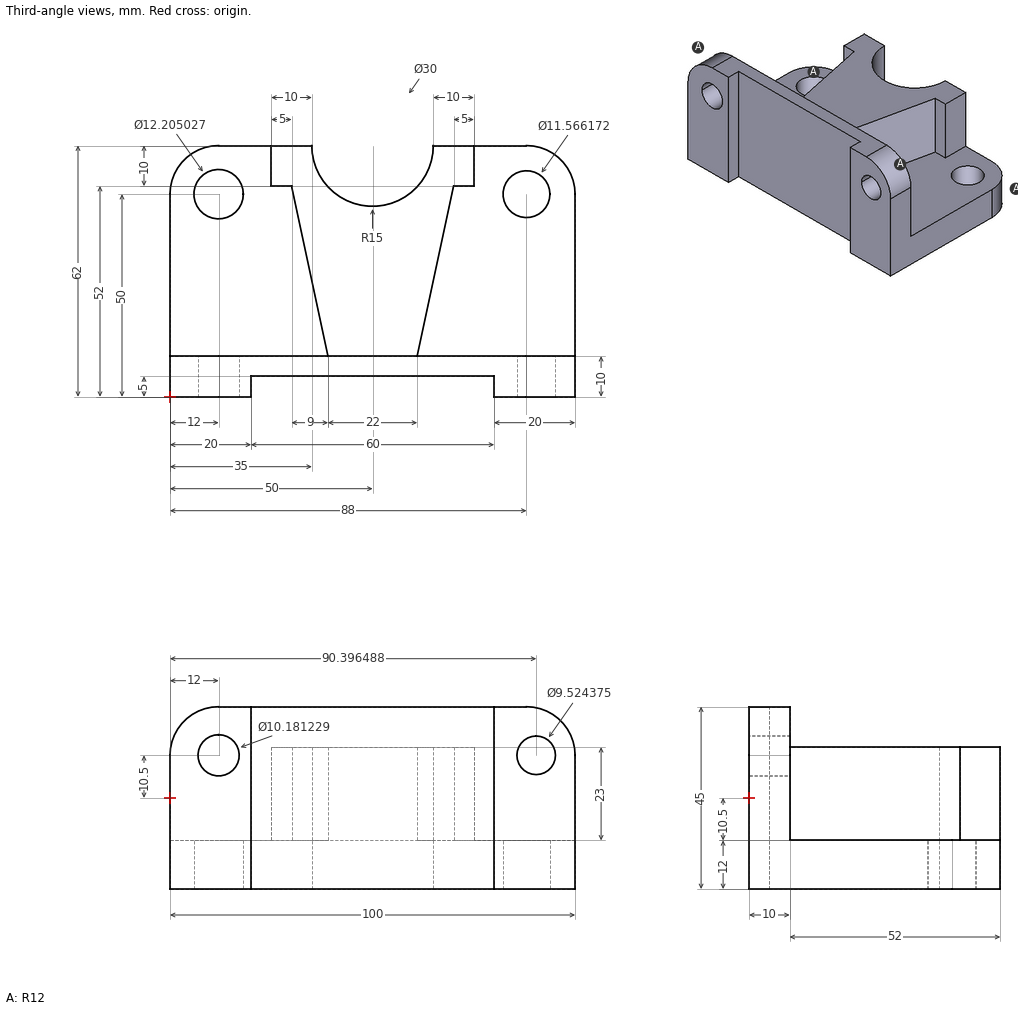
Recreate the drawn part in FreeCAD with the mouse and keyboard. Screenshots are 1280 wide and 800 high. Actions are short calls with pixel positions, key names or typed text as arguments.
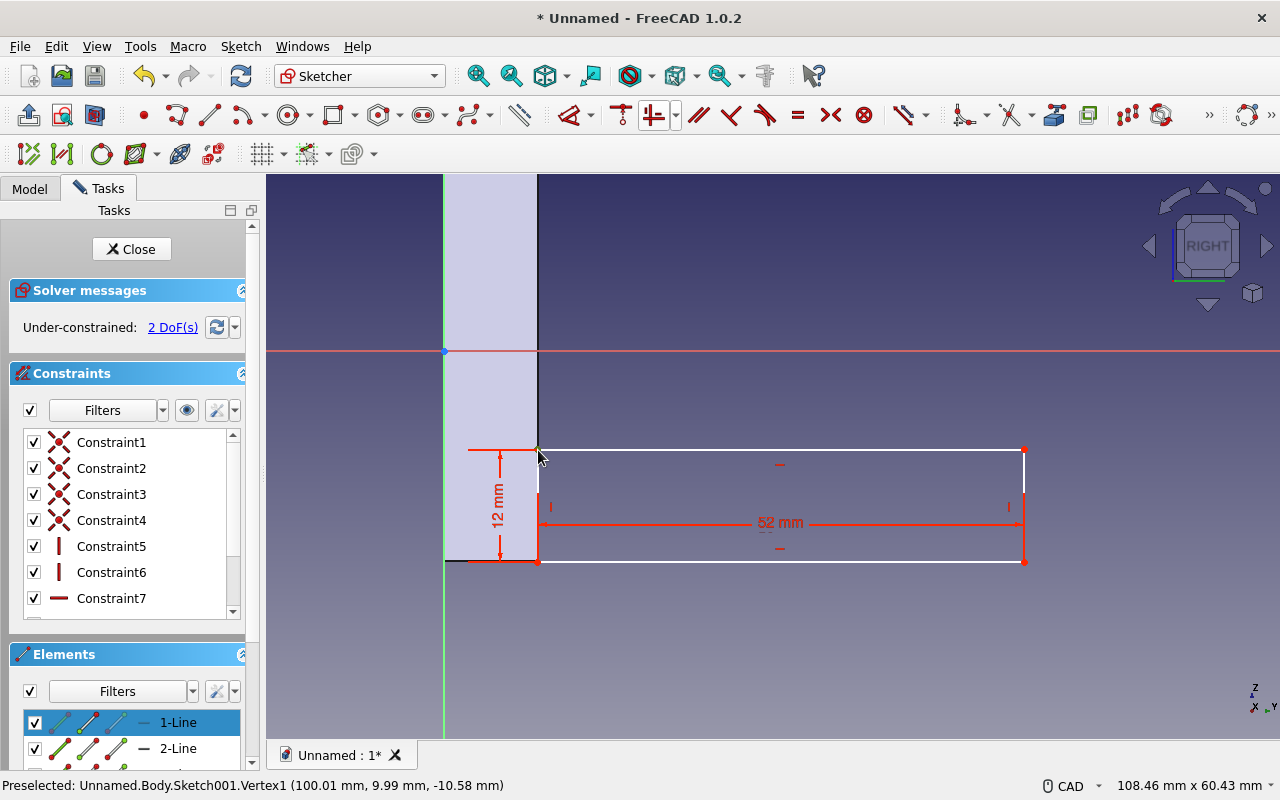
key(l)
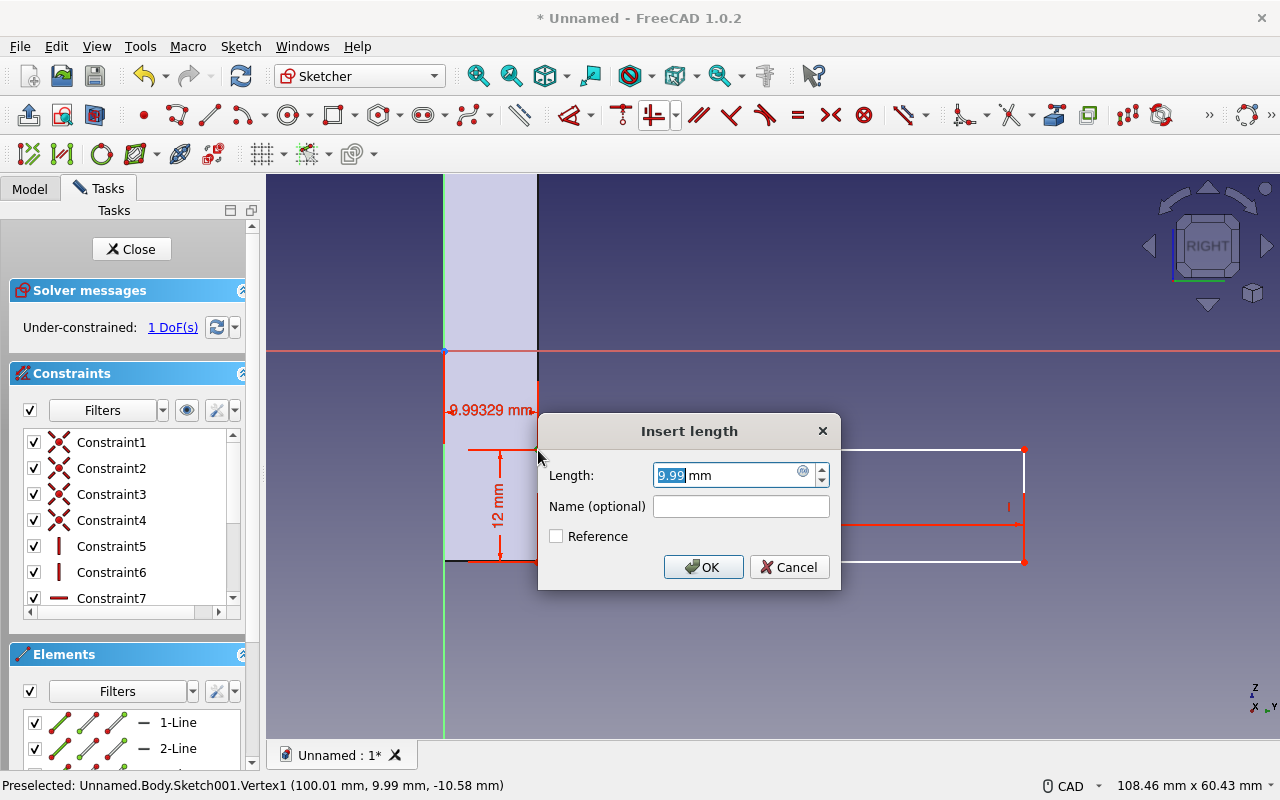
text(10)
key(Return)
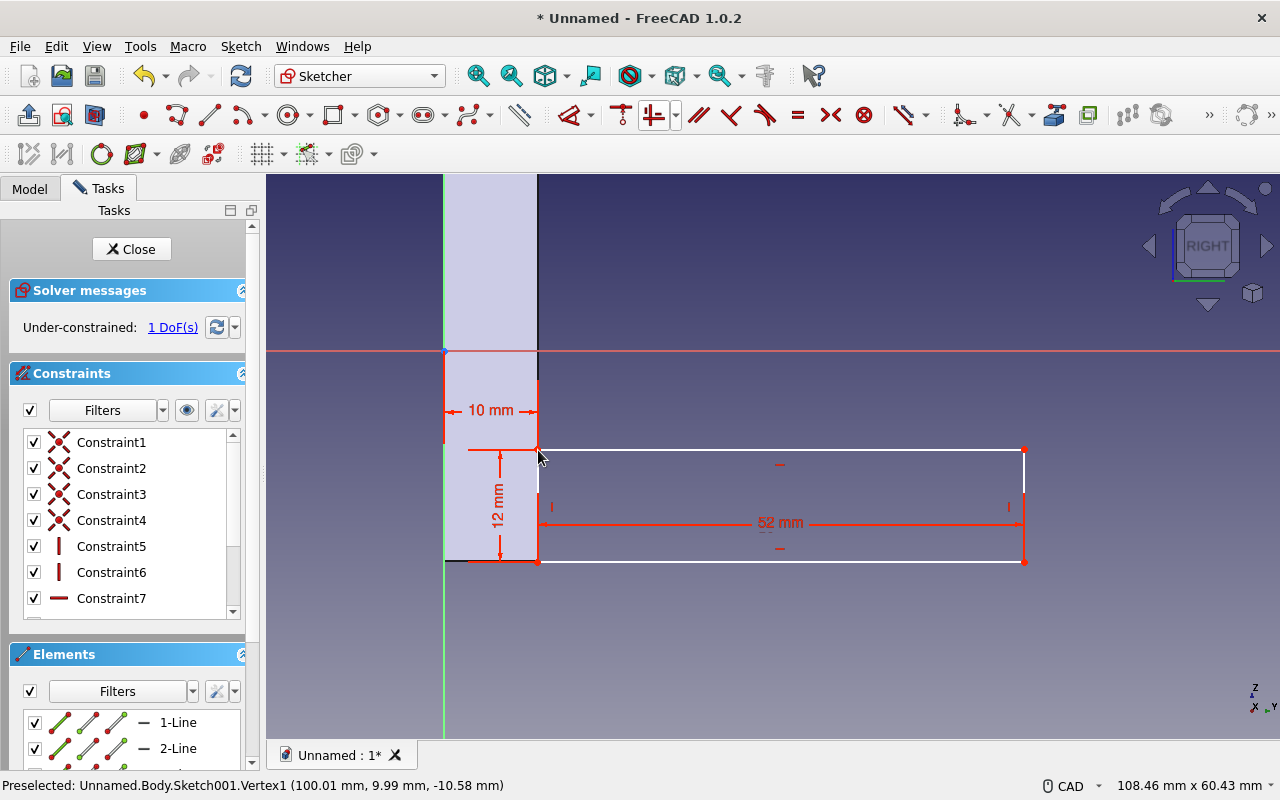
click(538, 450)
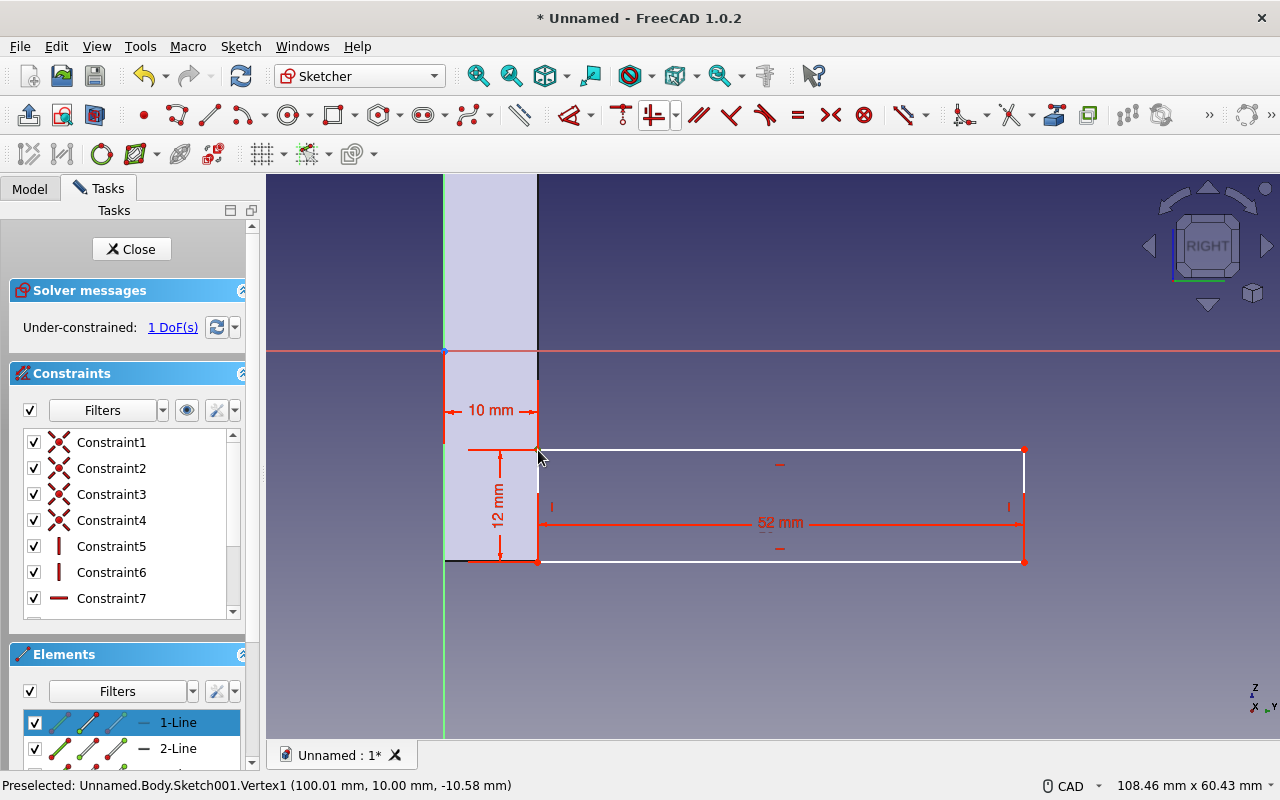
key(i)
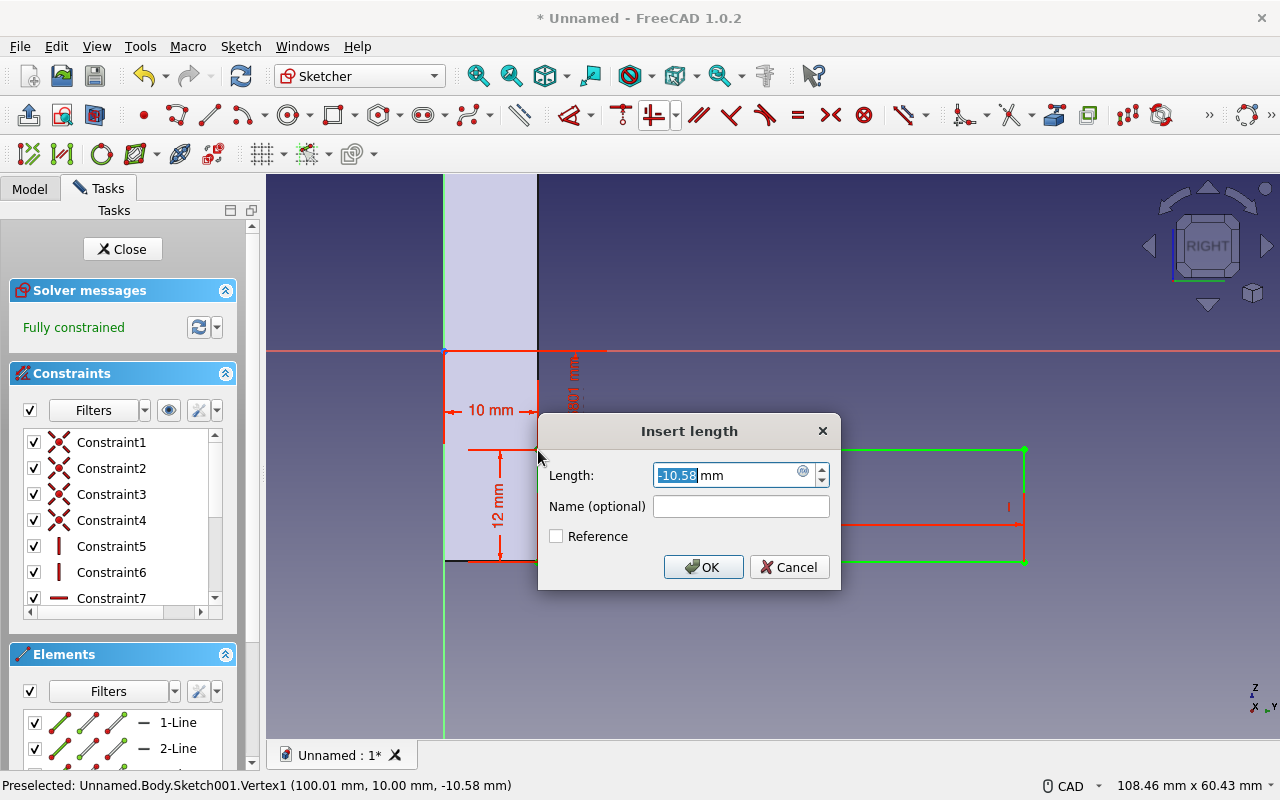
text(-10.5)
key(Return)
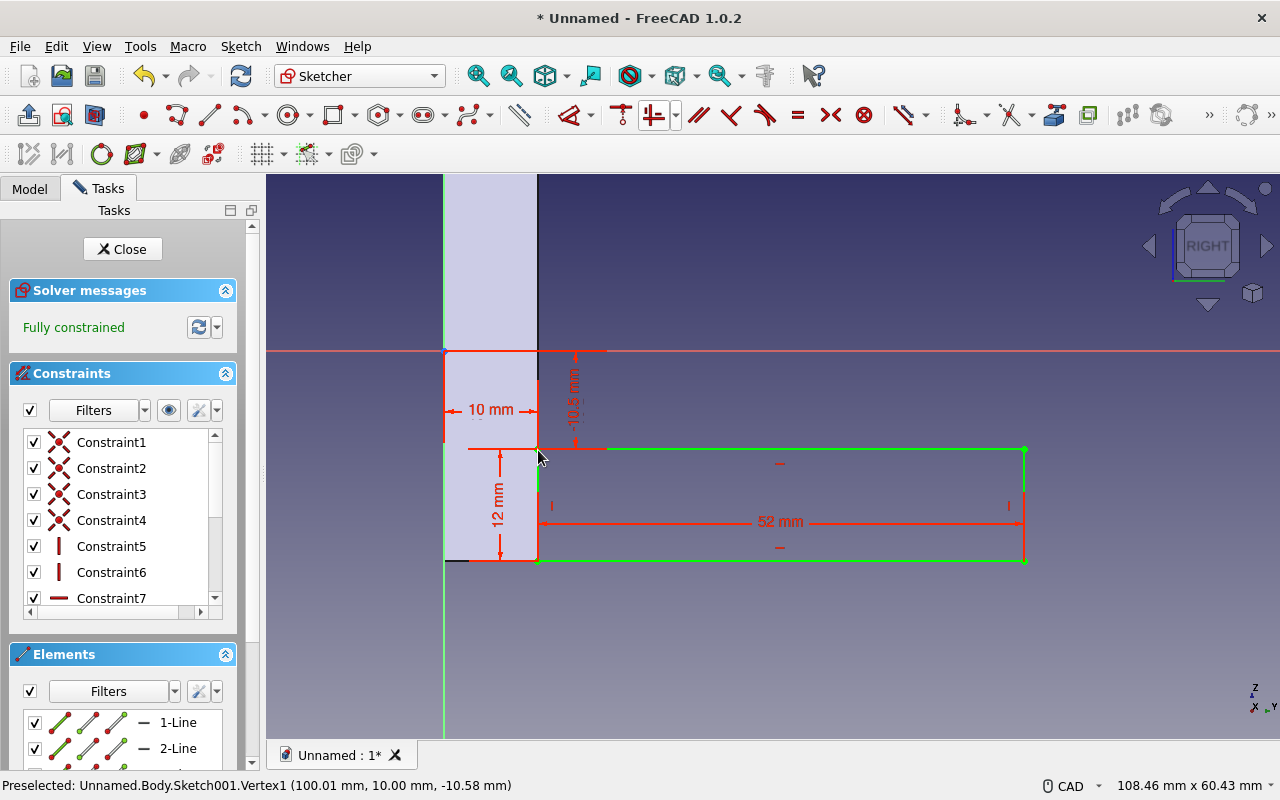
click(123, 249)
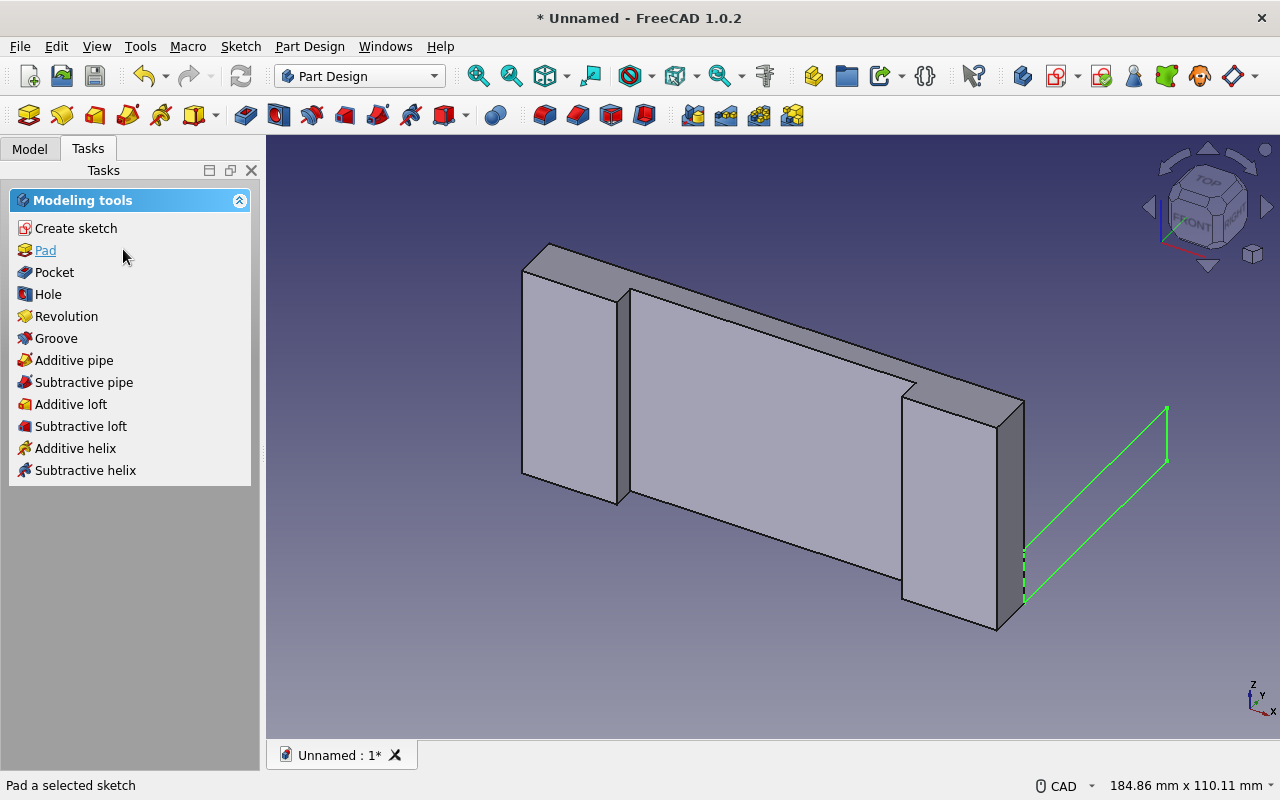
click(29, 116)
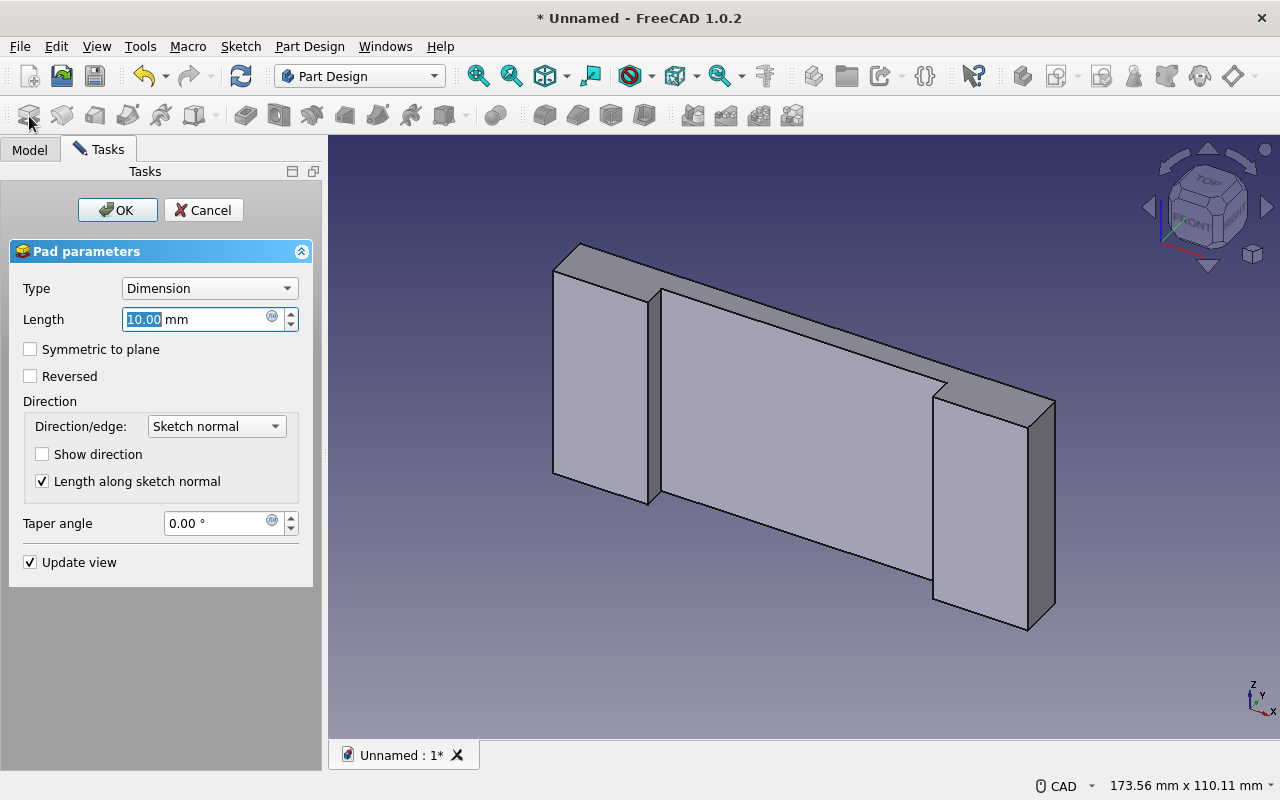
text(100)
key(Tab)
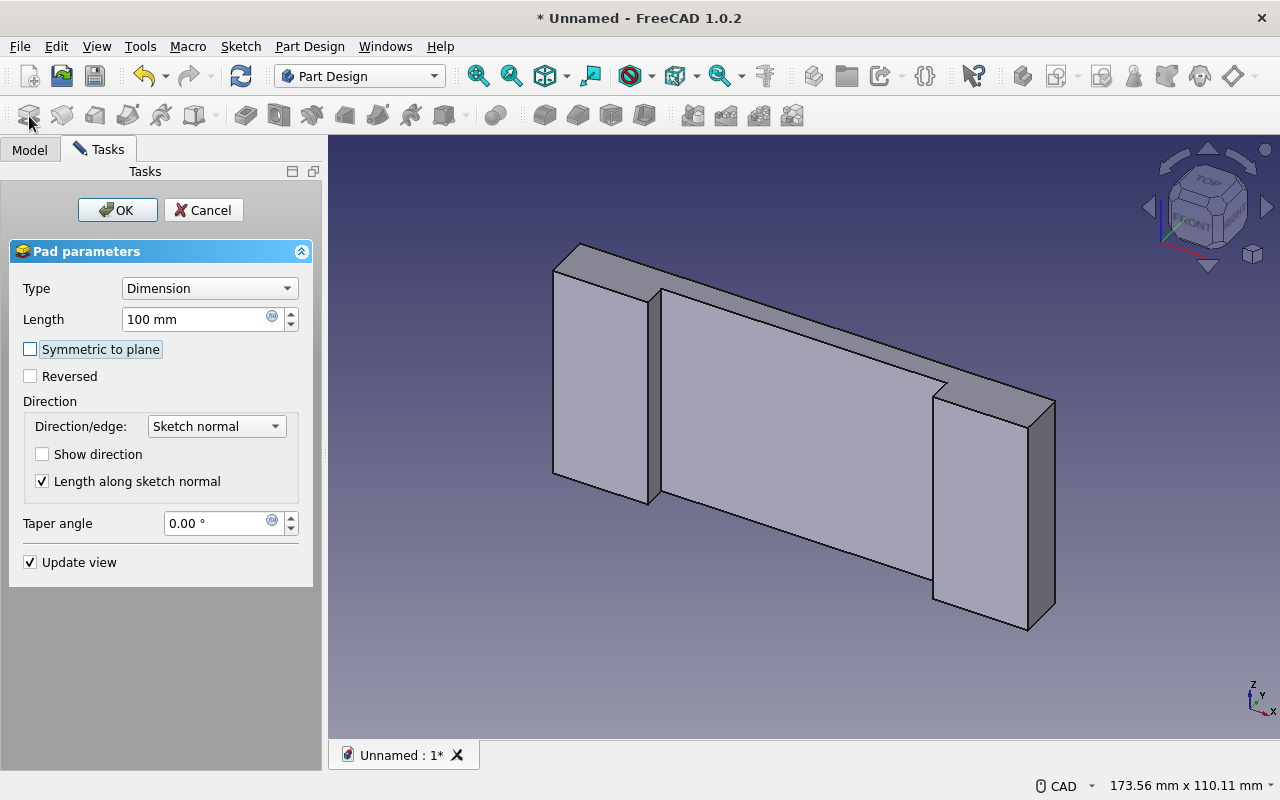
click(31, 376)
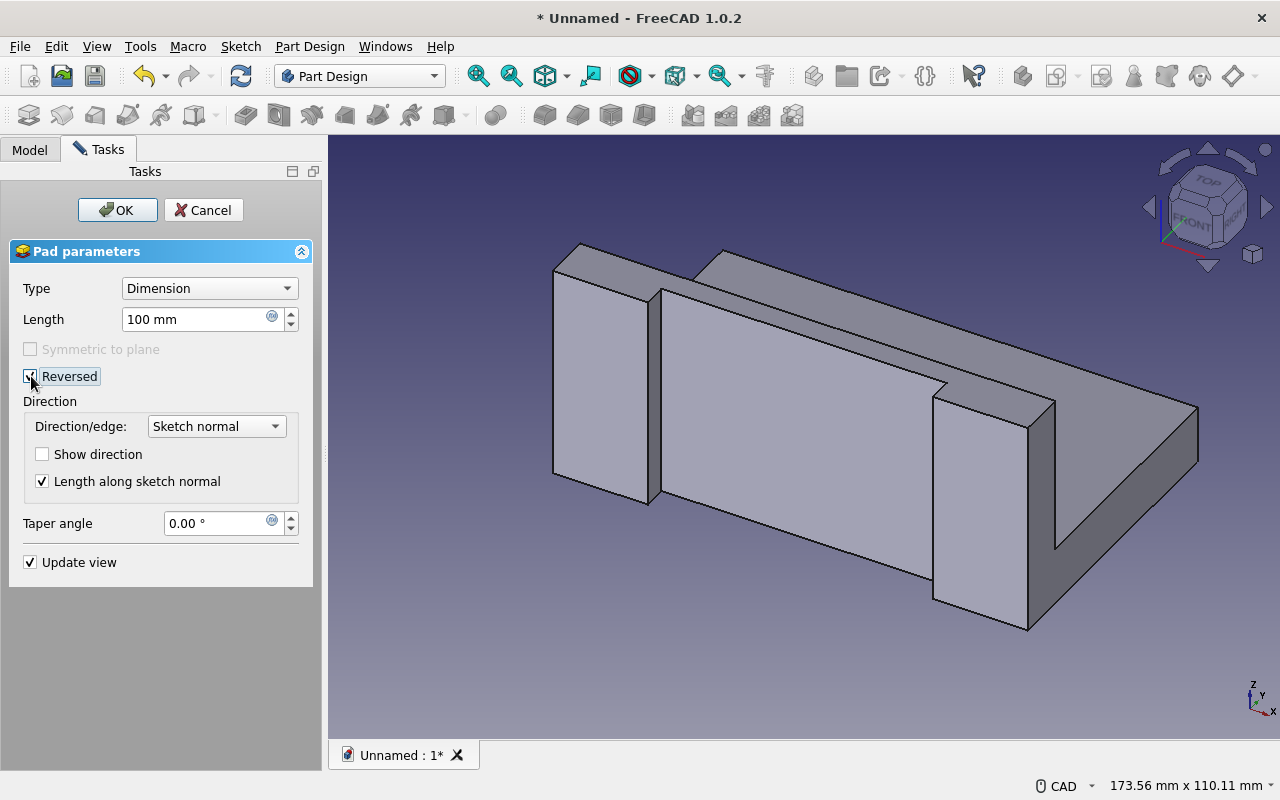
click(118, 210)